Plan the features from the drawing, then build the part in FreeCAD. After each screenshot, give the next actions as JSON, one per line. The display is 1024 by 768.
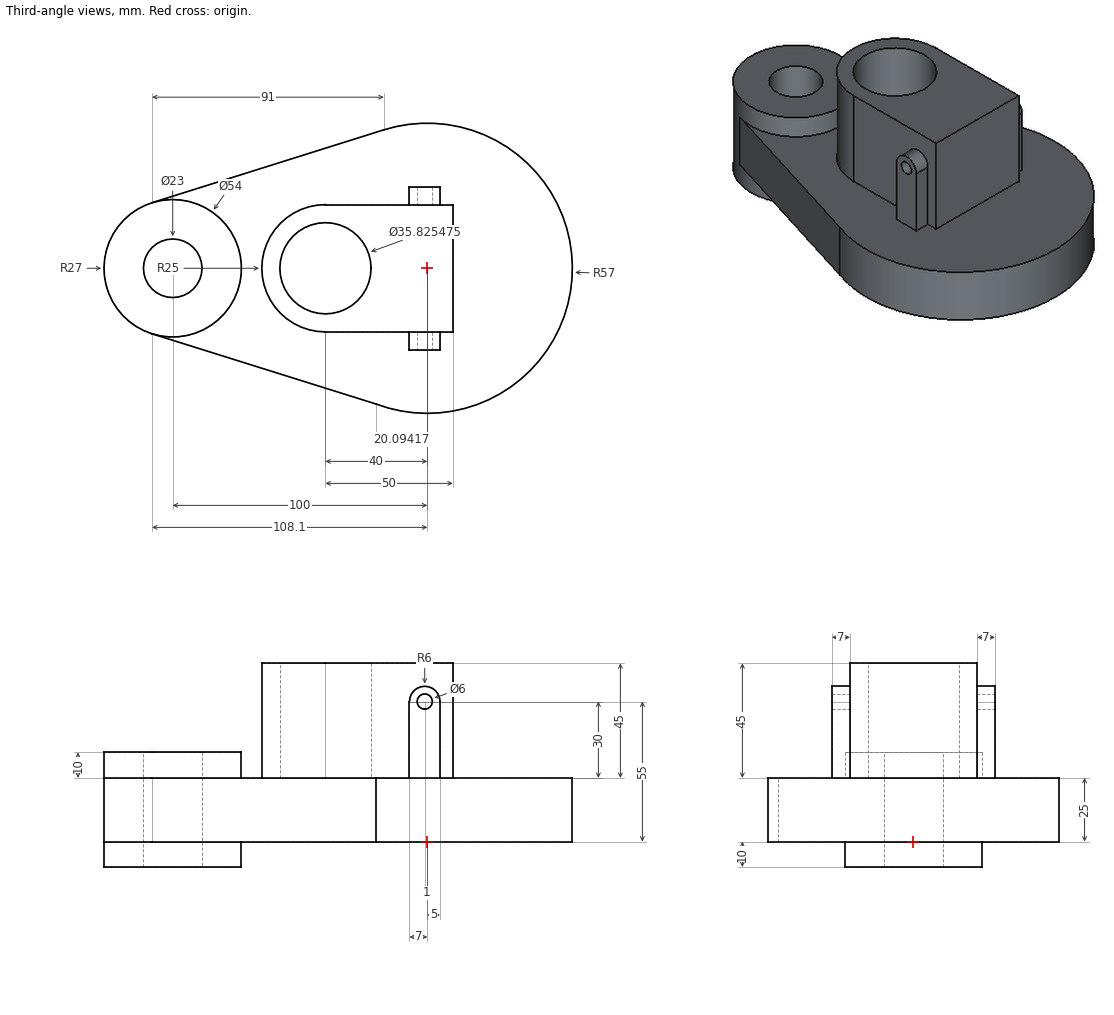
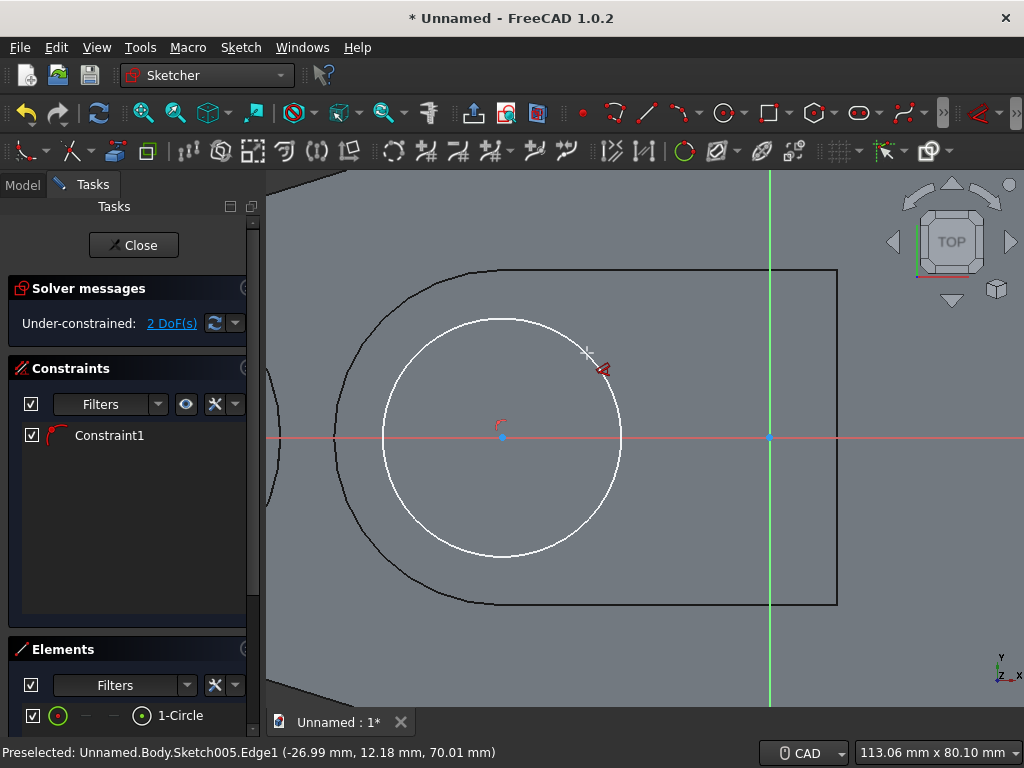
{"action": "left_click", "coordinate": [586, 353]}
{"action": "left_click", "coordinate": [609, 330]}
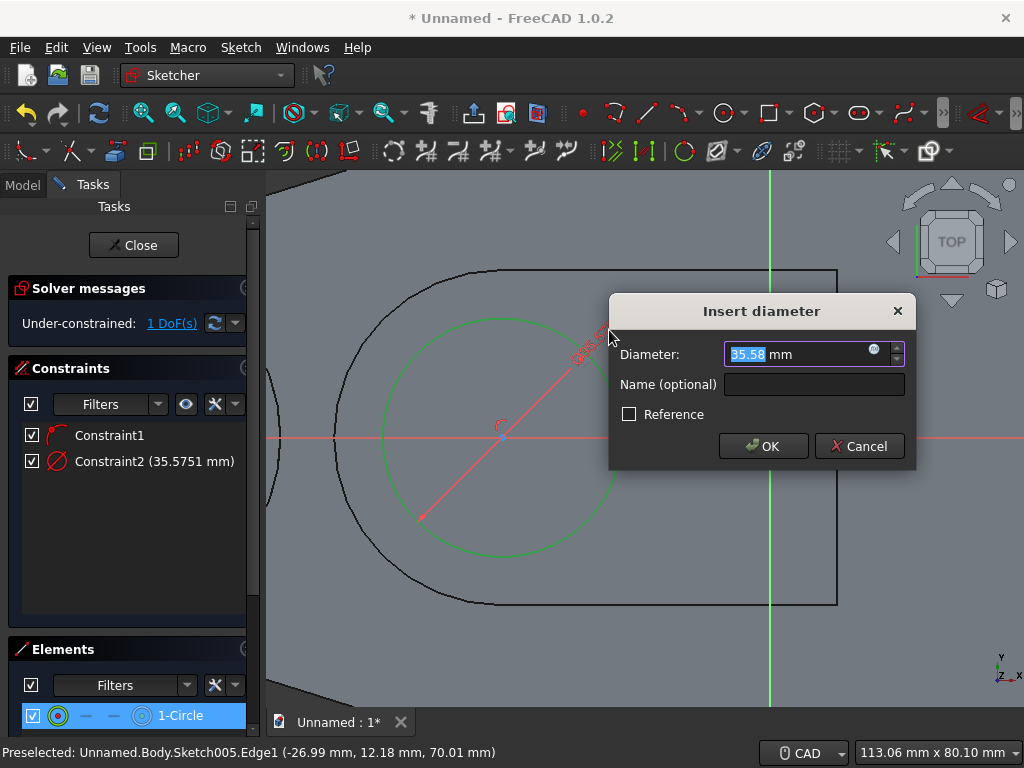
{"action": "type", "text": "35.825475"}
{"action": "key", "text": "Return"}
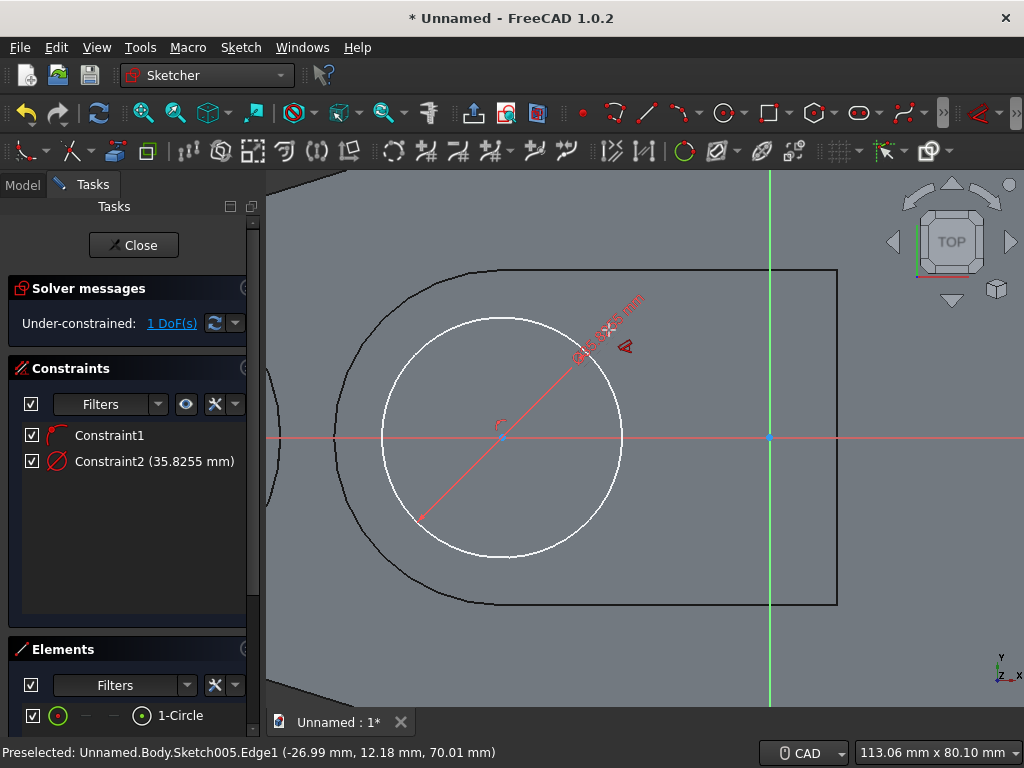
{"action": "left_click", "coordinate": [502, 438]}
{"action": "left_click", "coordinate": [636, 472]}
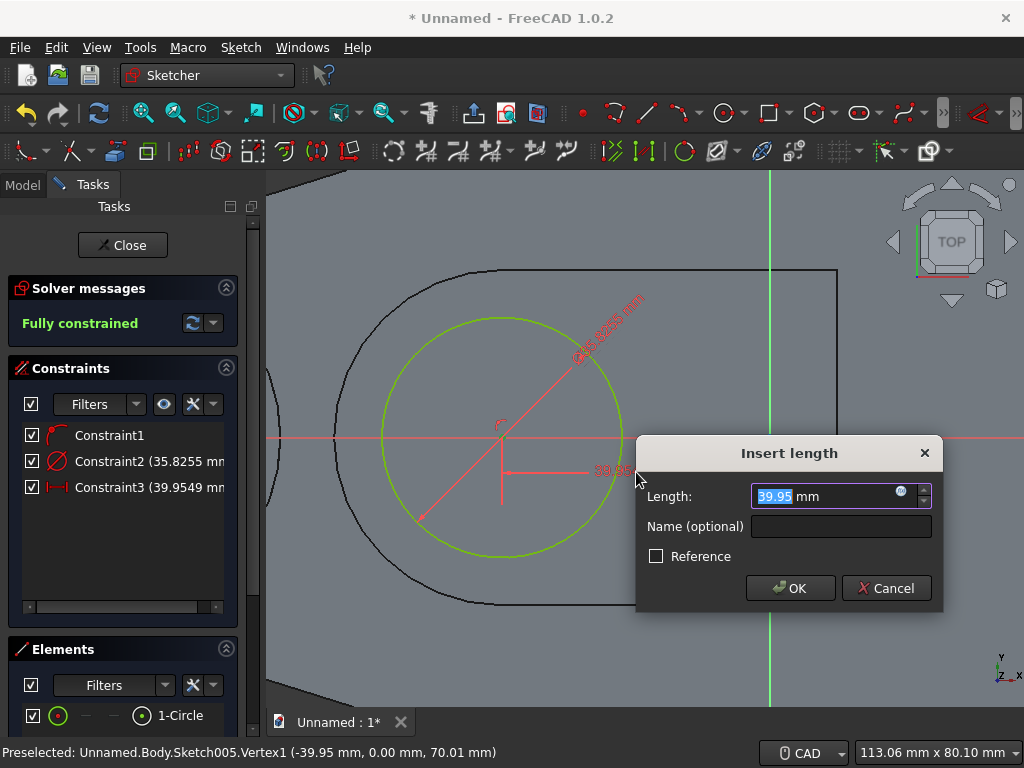
{"action": "type", "text": "40"}
{"action": "key", "text": "Return"}
{"action": "key", "text": "Escape"}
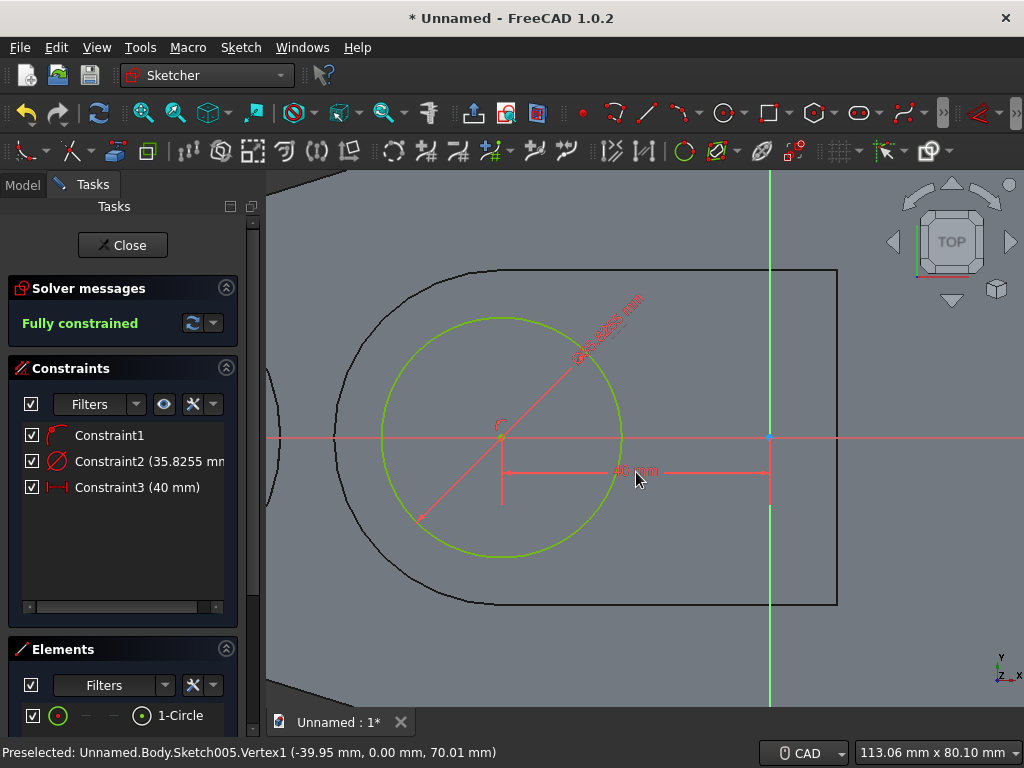
{"action": "left_click", "coordinate": [123, 245]}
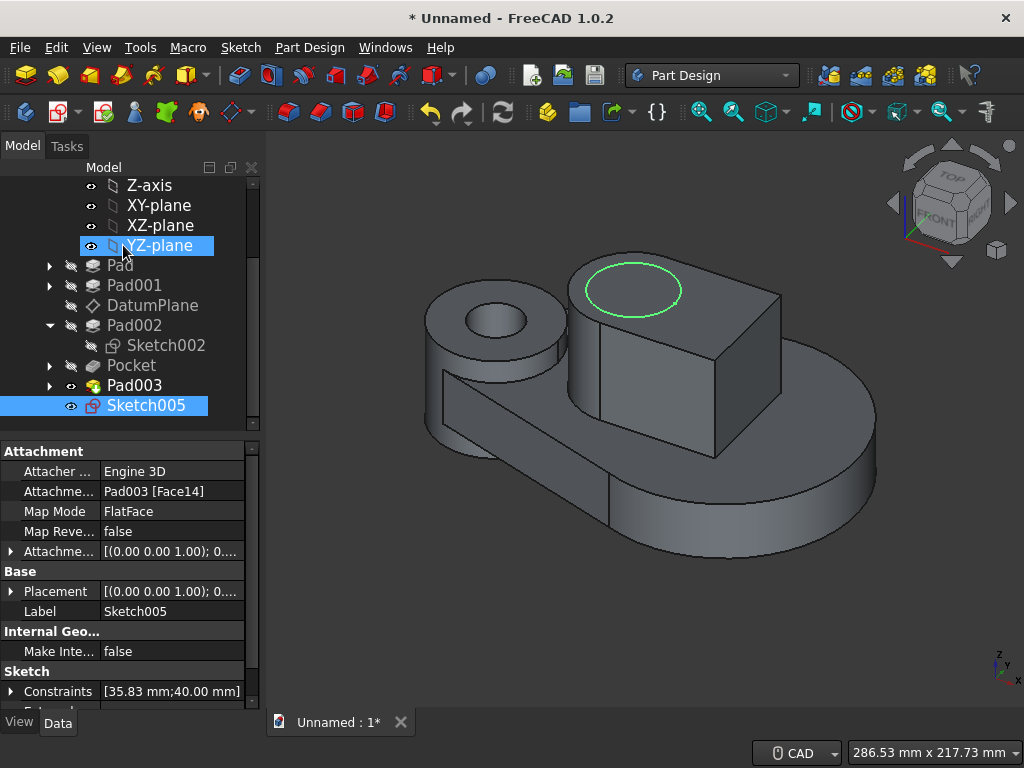
{"action": "left_click", "coordinate": [240, 76]}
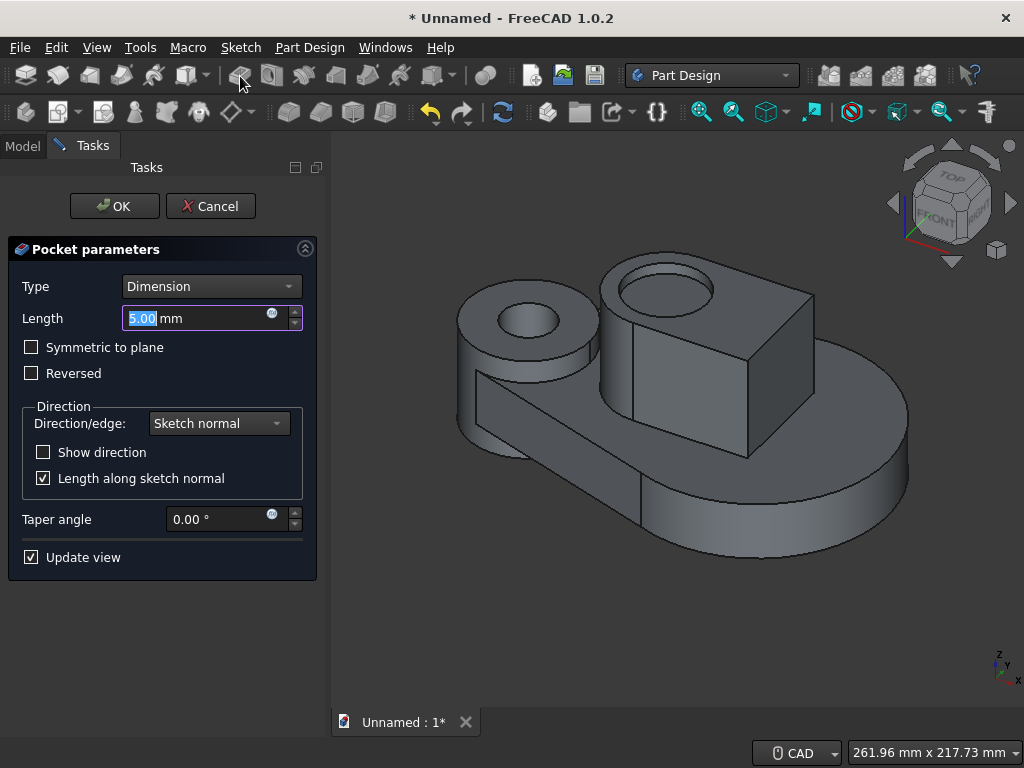
{"action": "type", "text": "45"}
{"action": "key", "text": "Tab"}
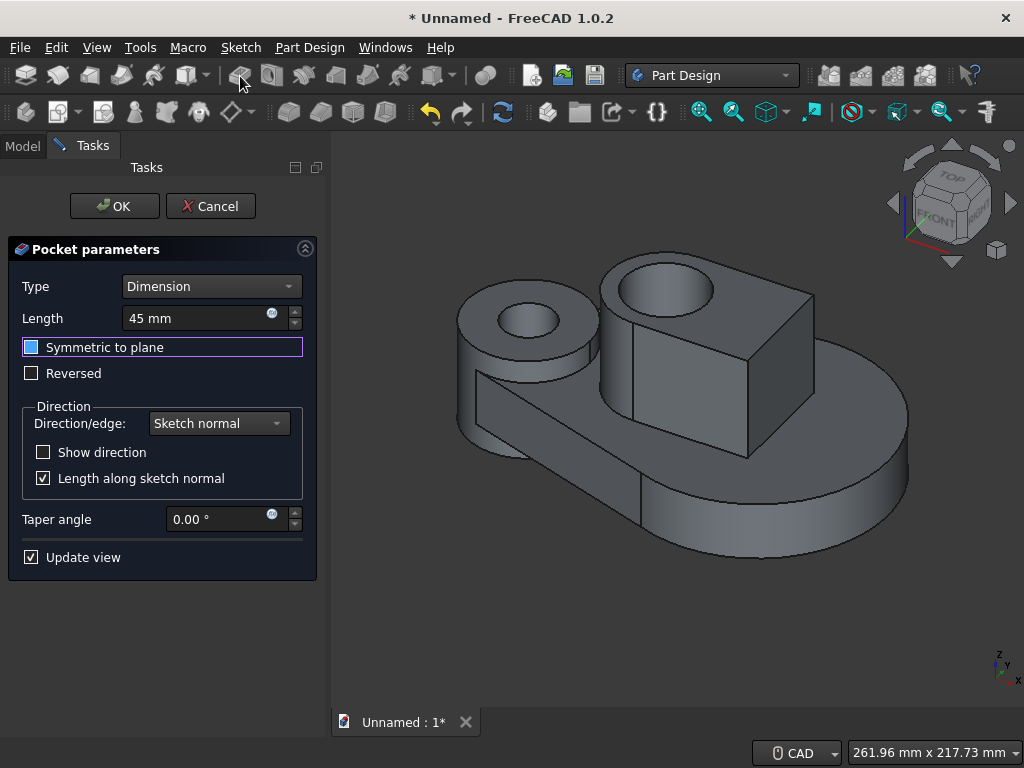
{"action": "left_click", "coordinate": [115, 206]}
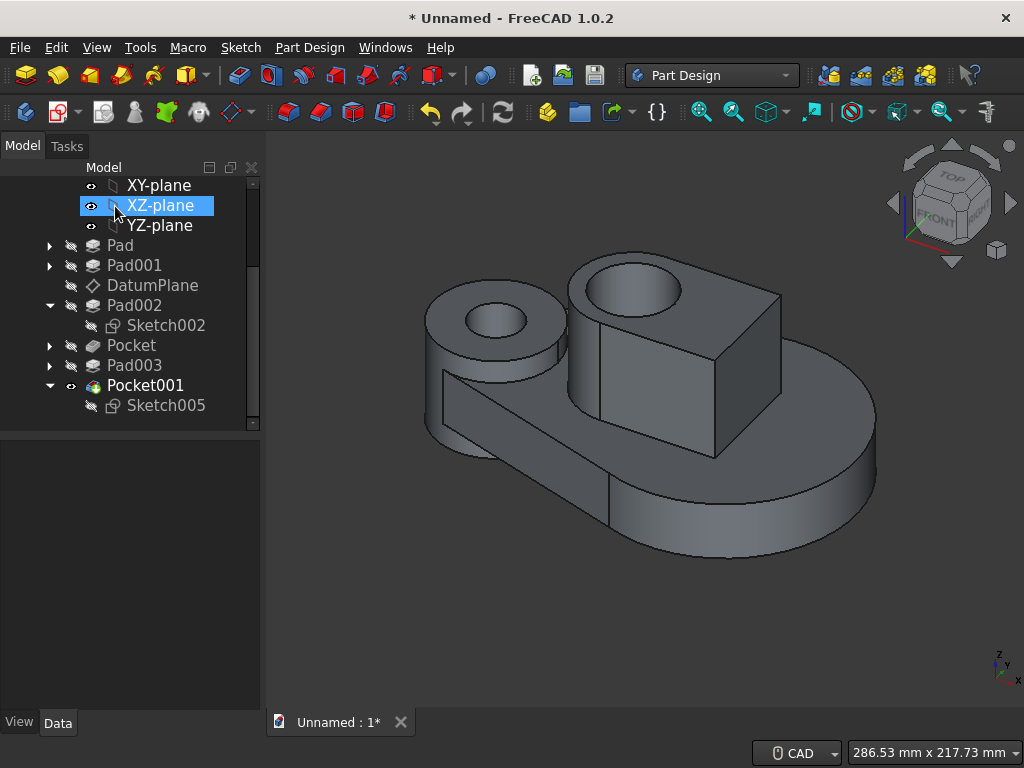
{"action": "left_click", "coordinate": [658, 390]}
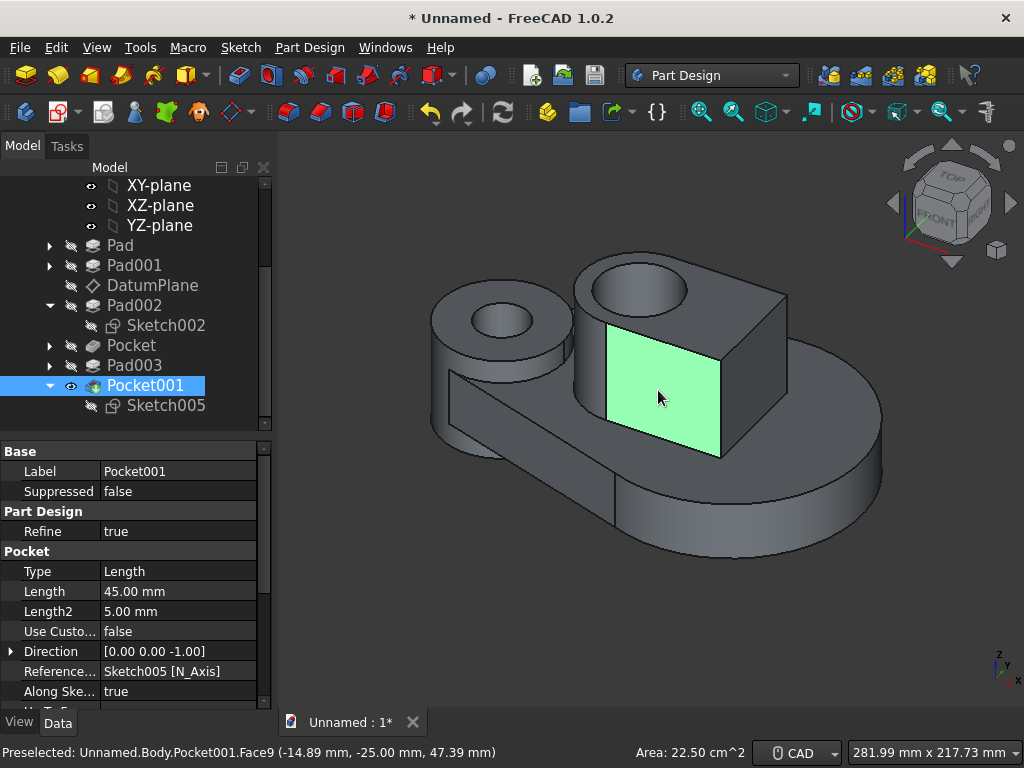
{"action": "left_click", "coordinate": [58, 112]}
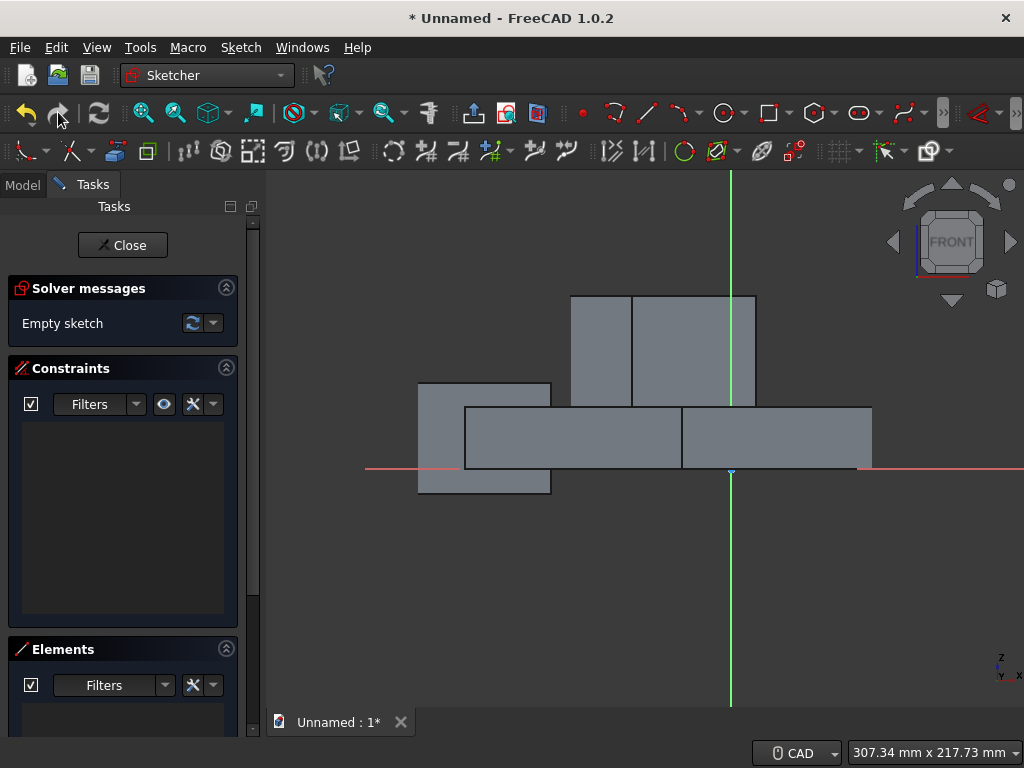
{"action": "scroll", "coordinate": [853, 357], "scroll_direction": "up", "scroll_amount": 4}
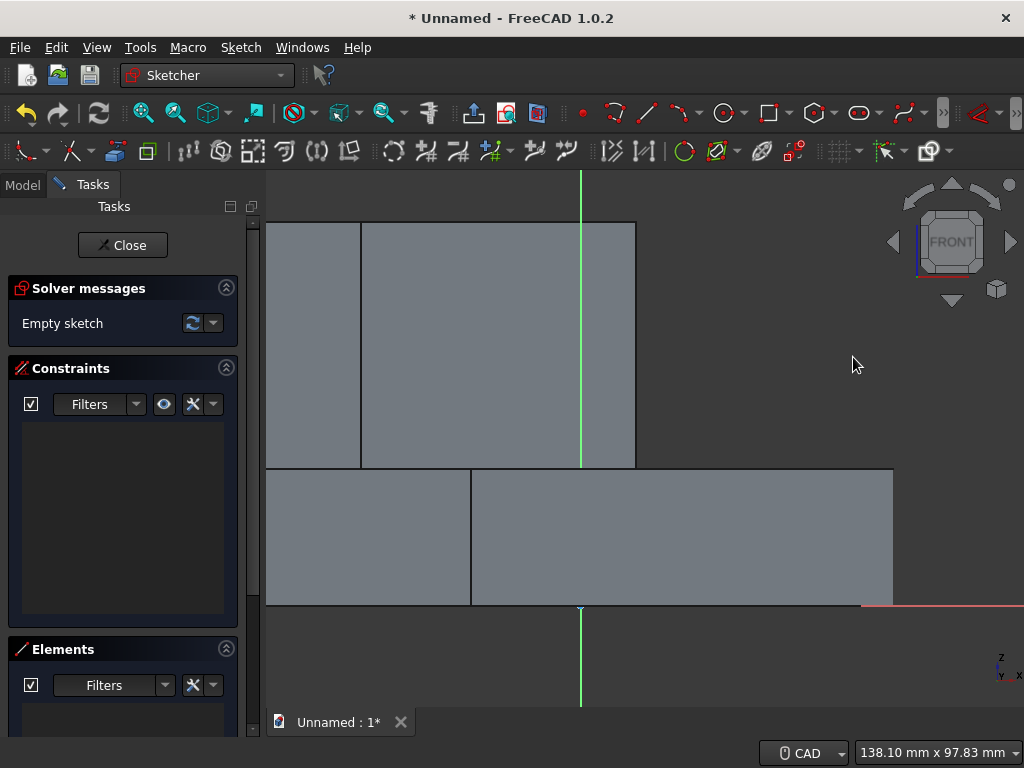
{"action": "key", "text": "g m"}